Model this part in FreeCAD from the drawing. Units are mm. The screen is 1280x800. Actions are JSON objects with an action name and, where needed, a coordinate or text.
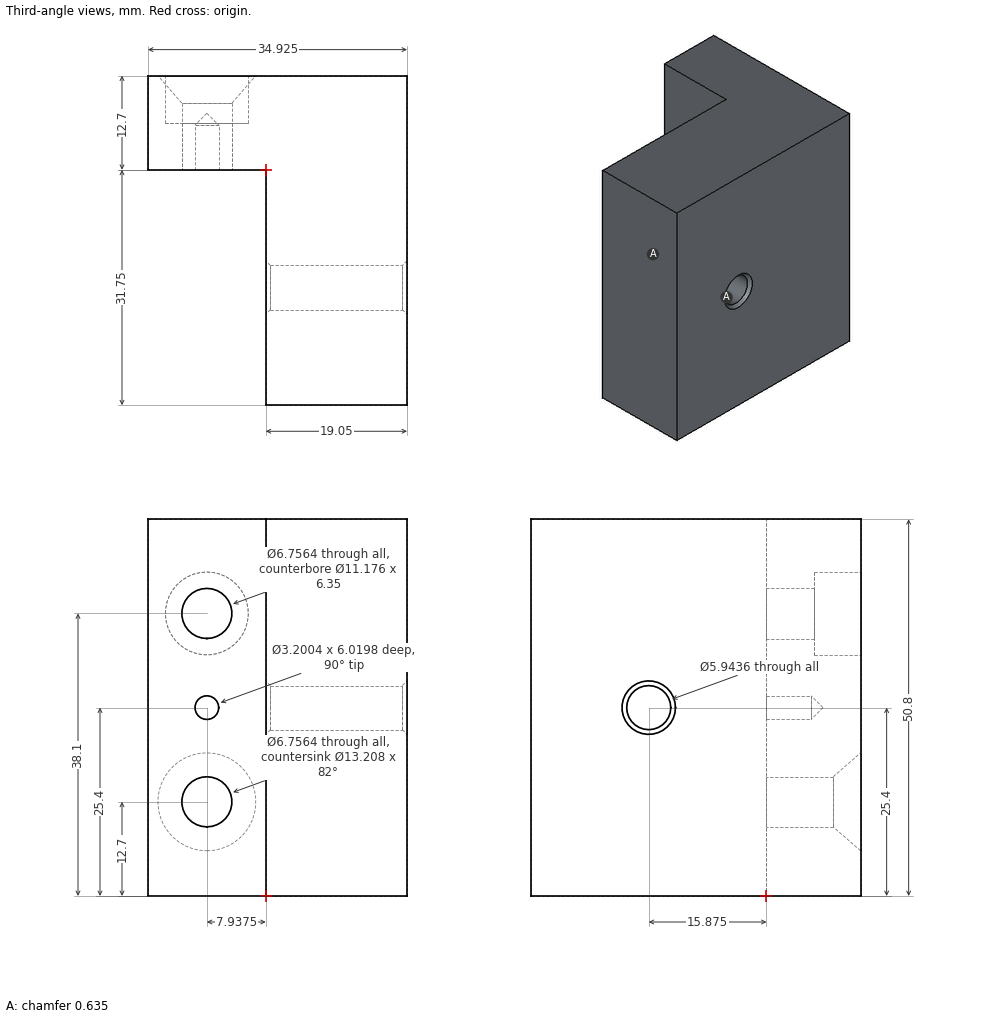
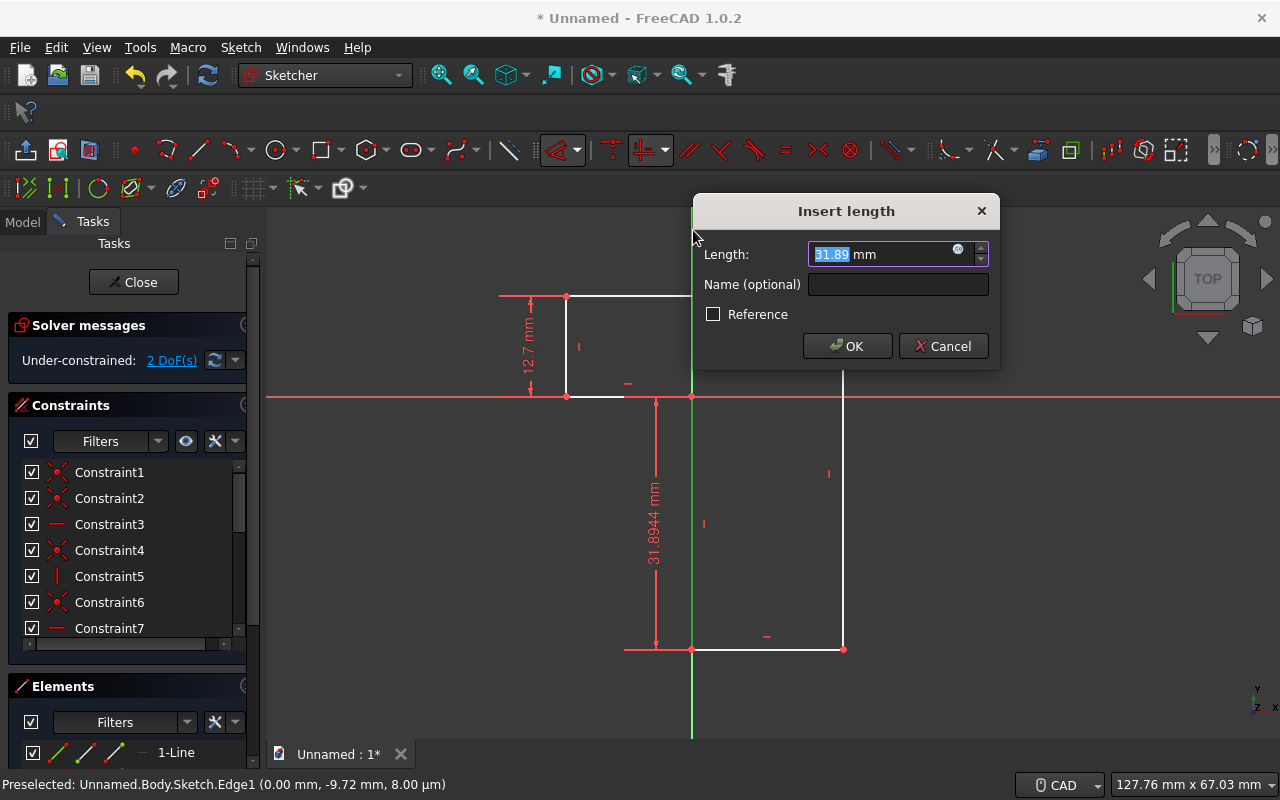
{"action": "type", "text": "31.75"}
{"action": "key", "text": "Return"}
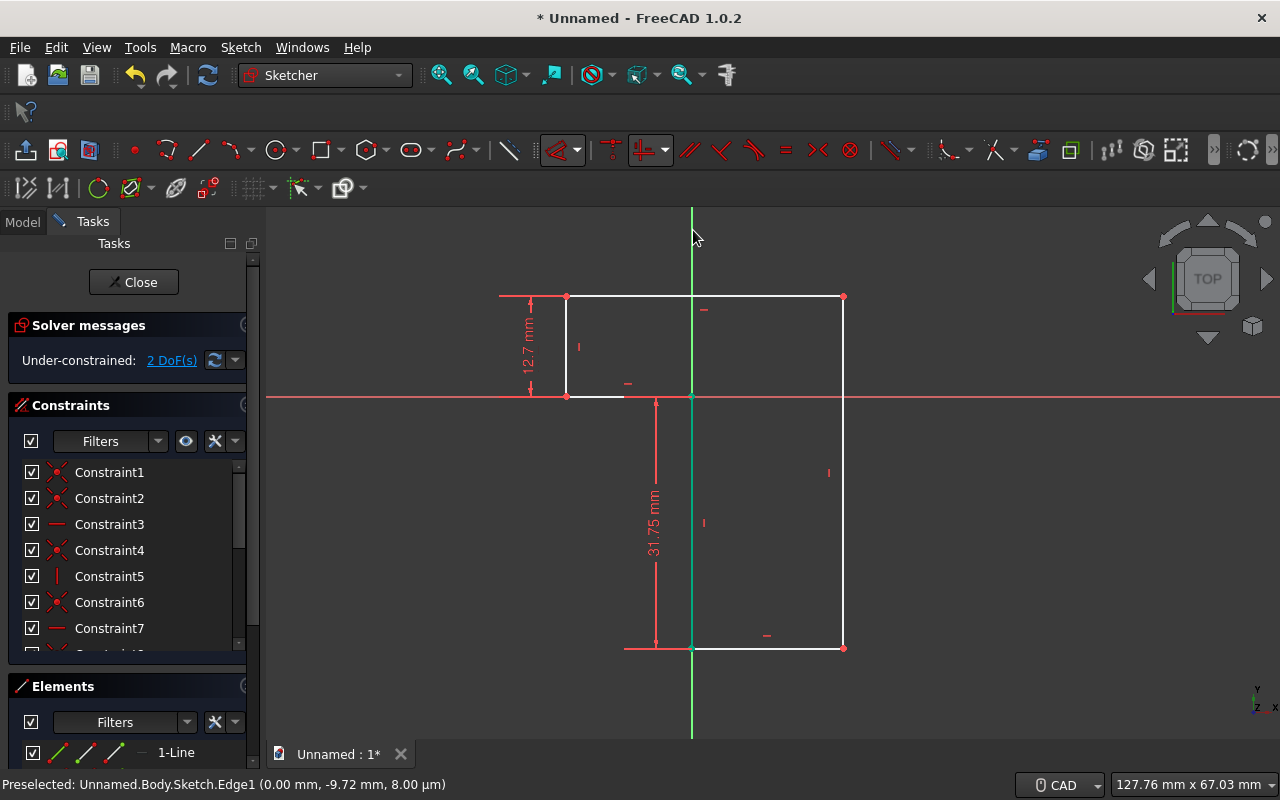
{"action": "left_click", "coordinate": [737, 649]}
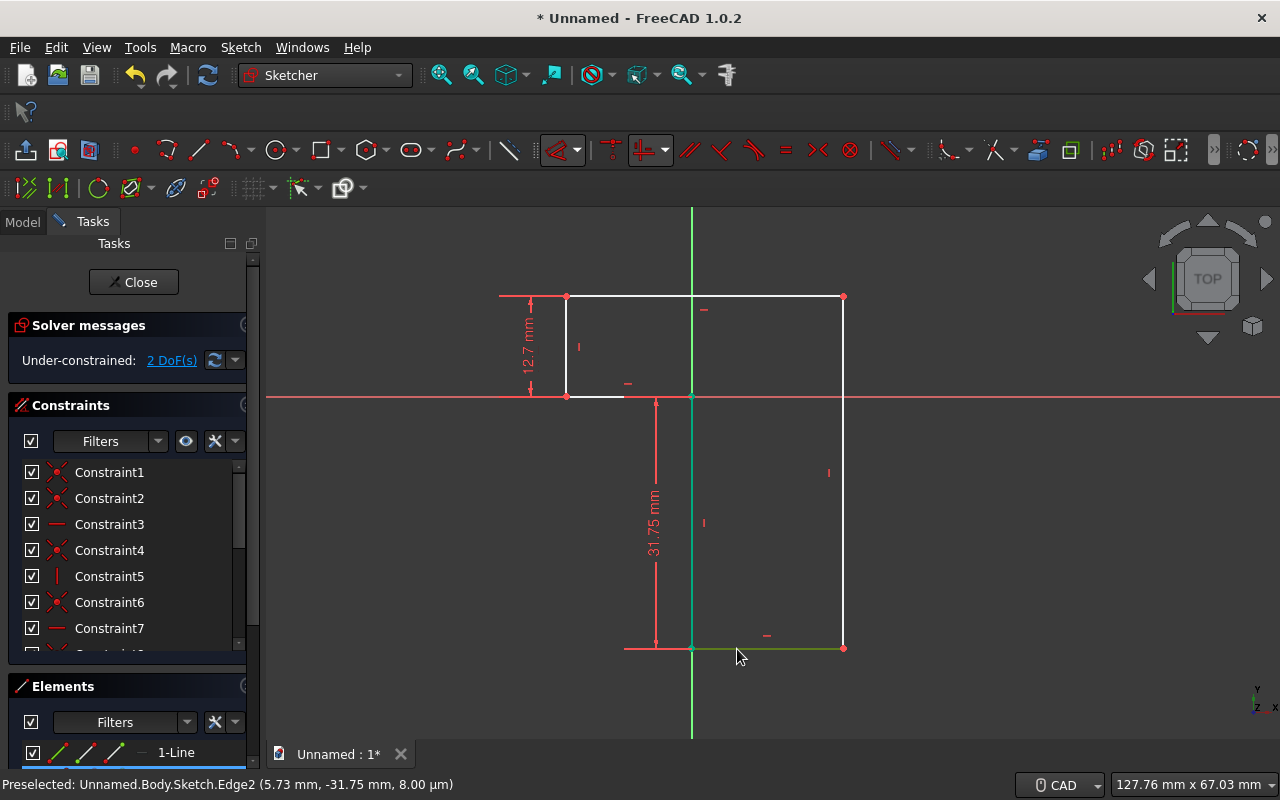
{"action": "key", "text": "l"}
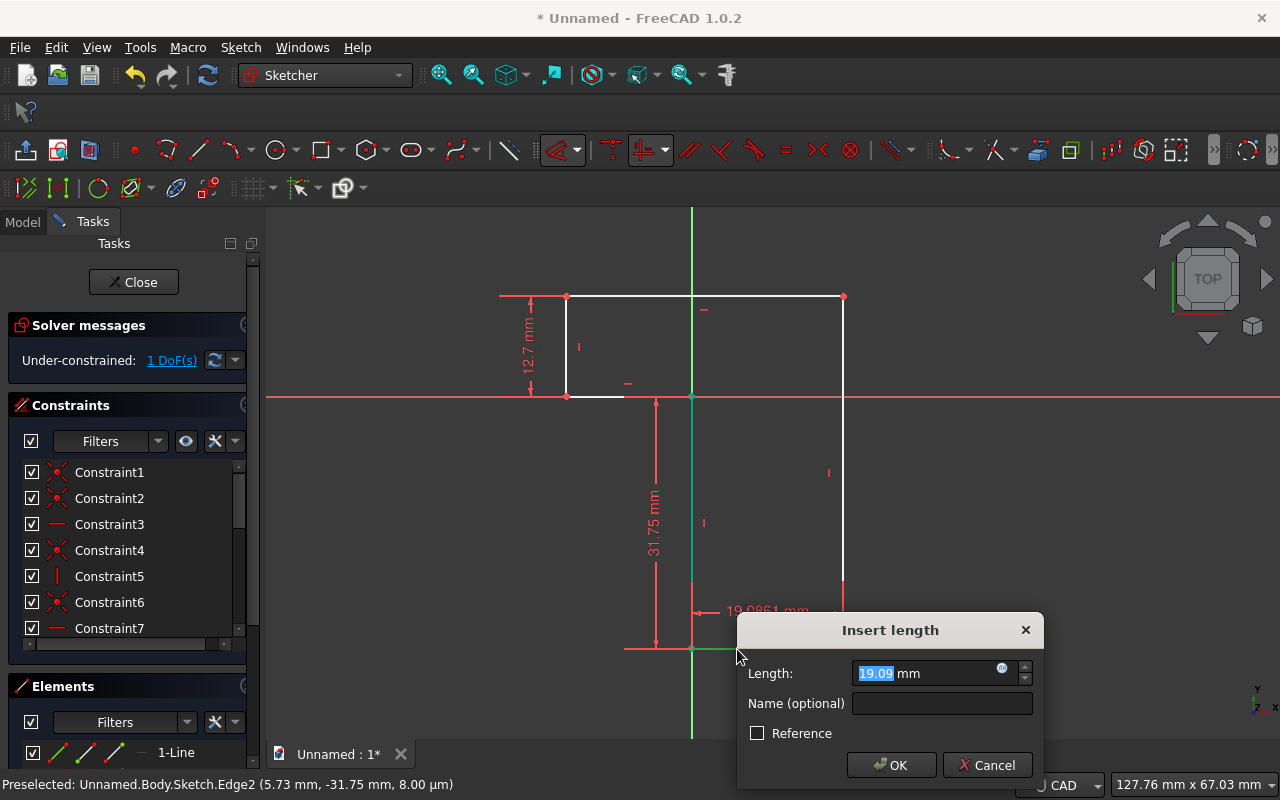
{"action": "type", "text": "19.05"}
{"action": "key", "text": "Return"}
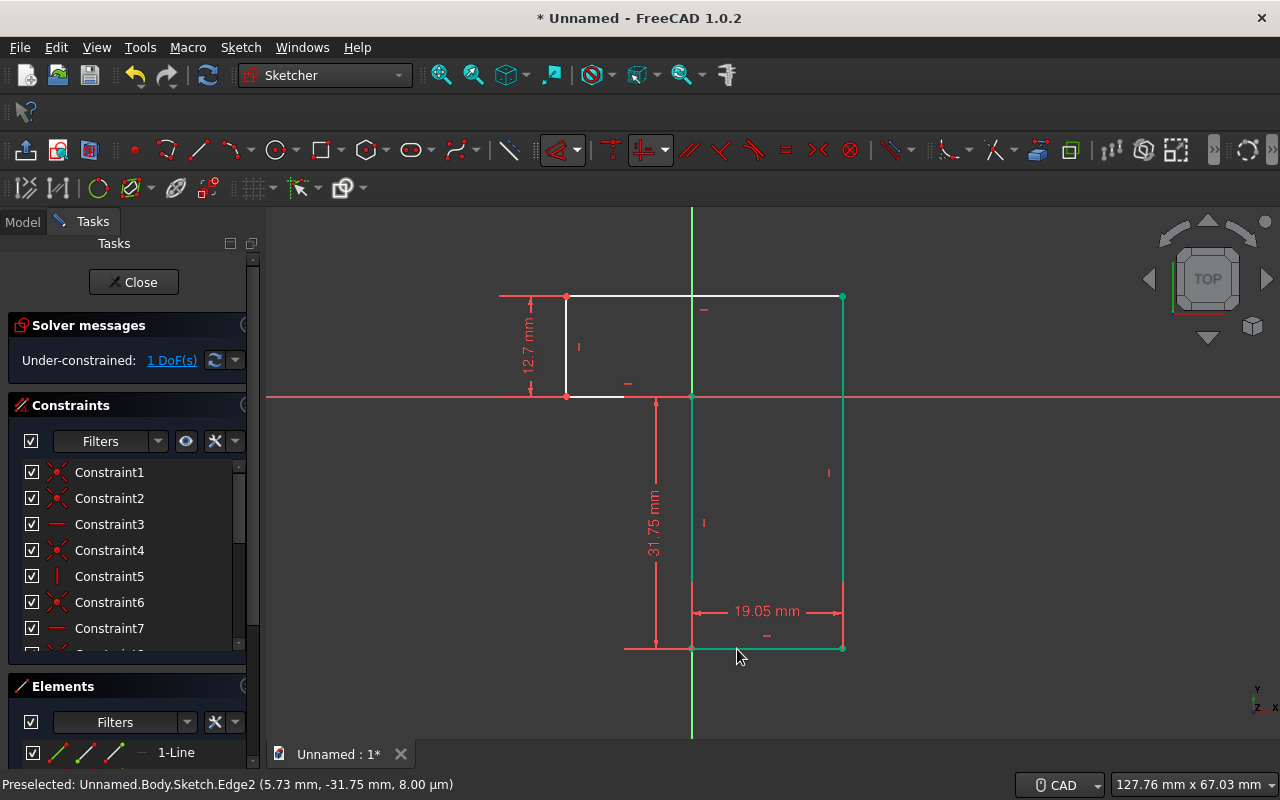
{"action": "left_click", "coordinate": [760, 296]}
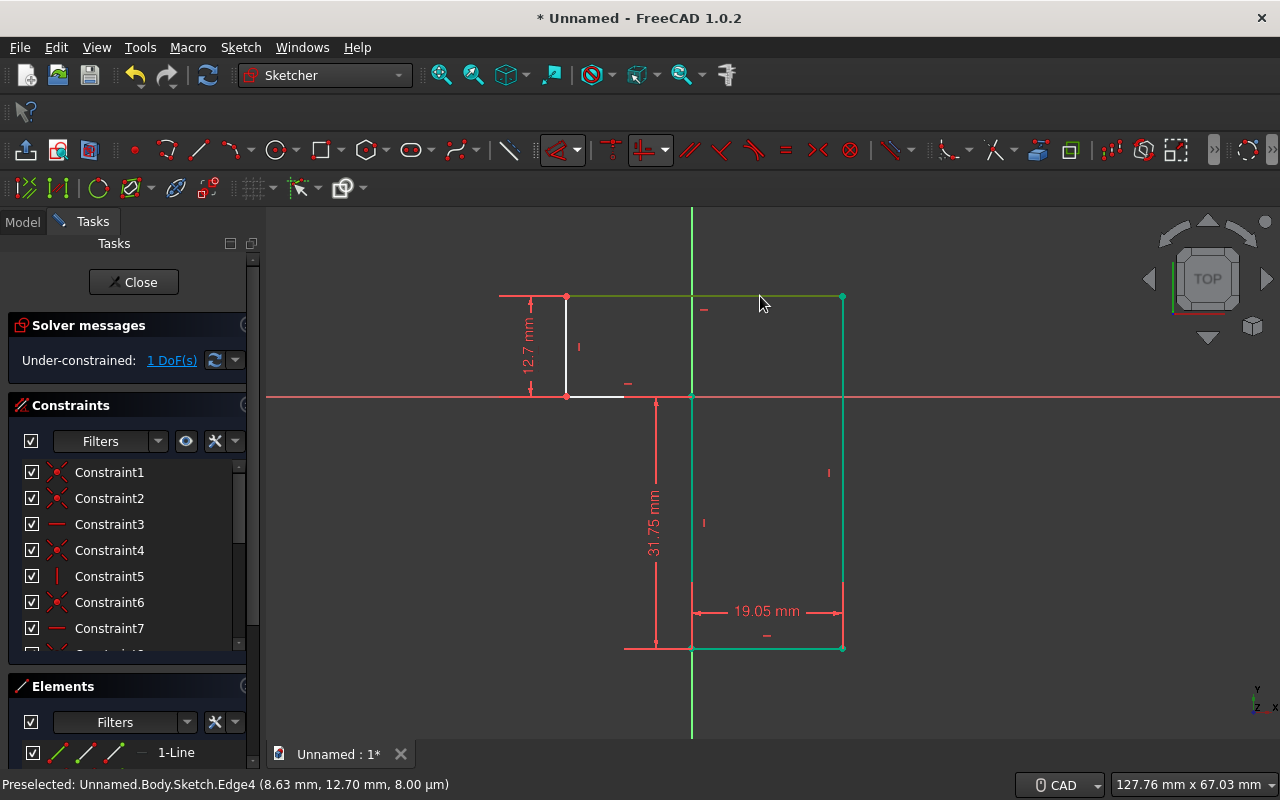
{"action": "left_click", "coordinate": [580, 150]}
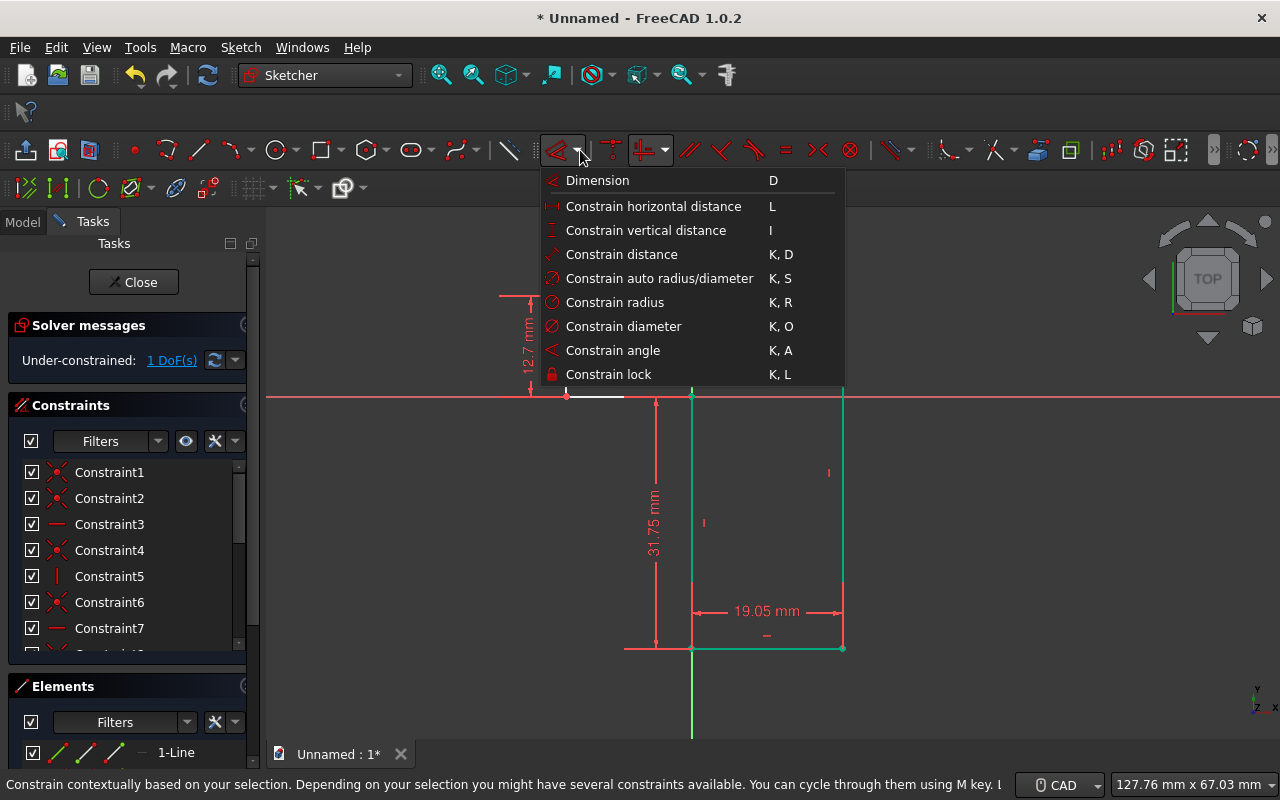
{"action": "left_click", "coordinate": [693, 206]}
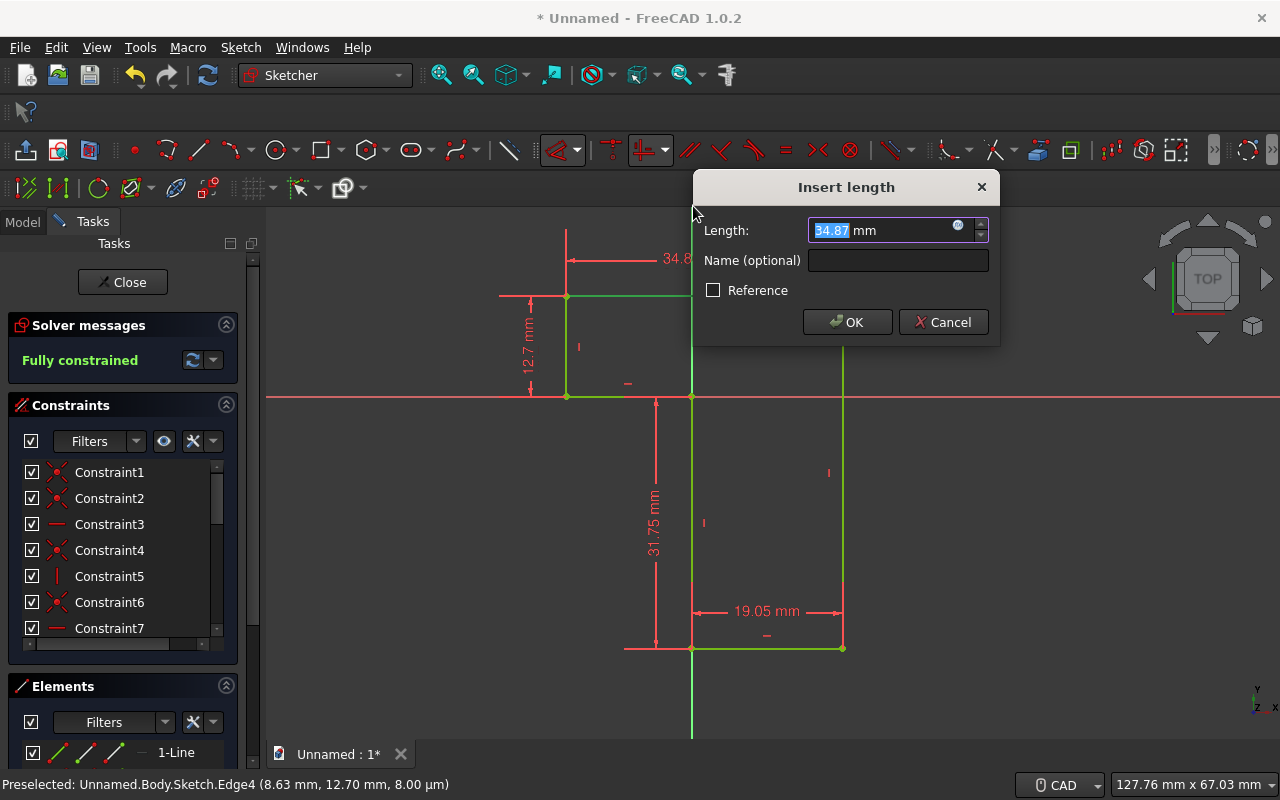
{"action": "type", "text": "34.925"}
{"action": "key", "text": "Return"}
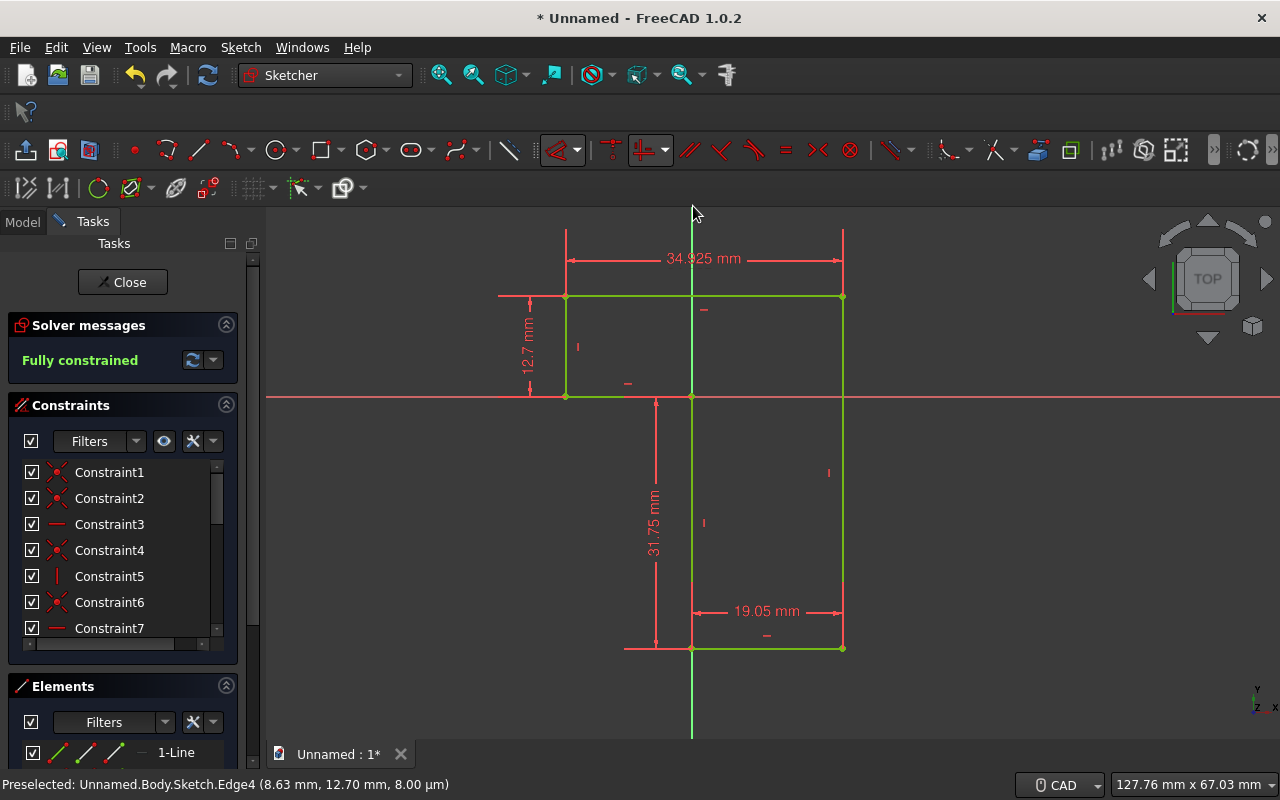
{"action": "left_click", "coordinate": [123, 282]}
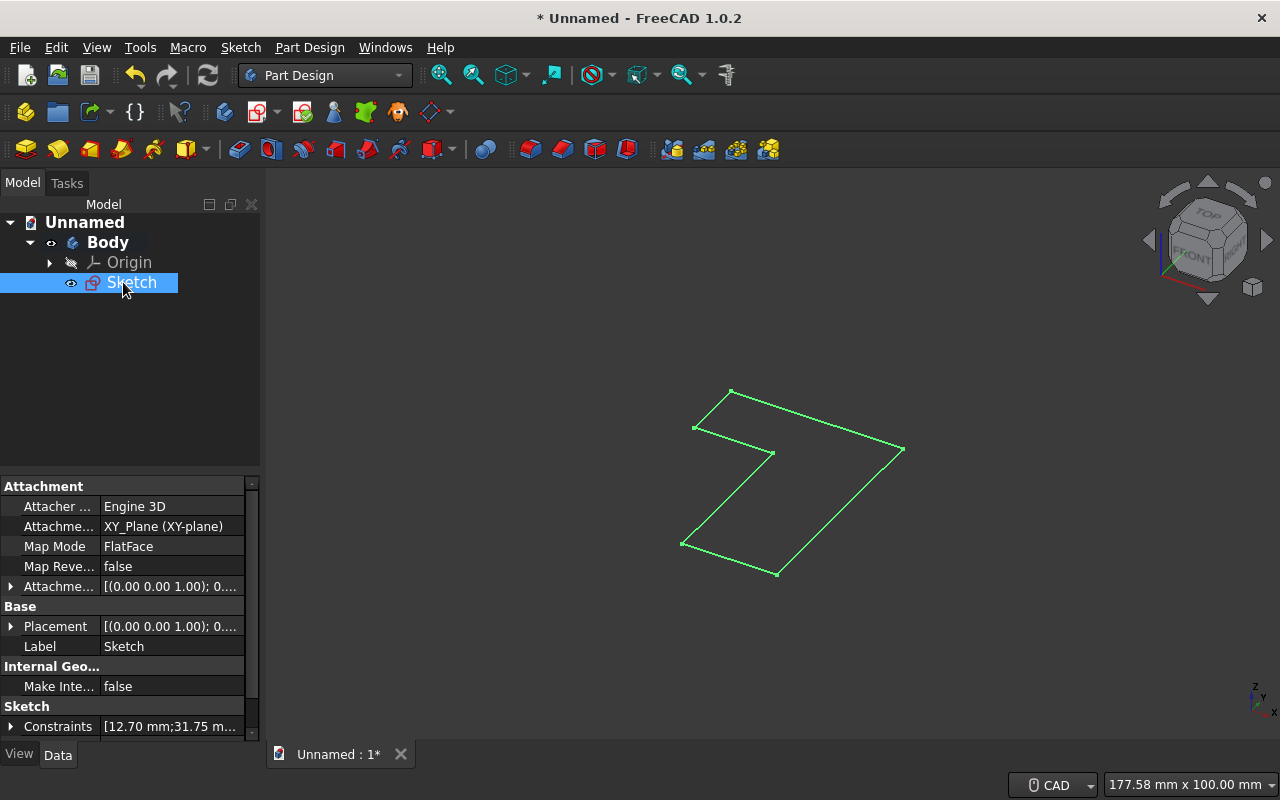
{"action": "left_click", "coordinate": [26, 150]}